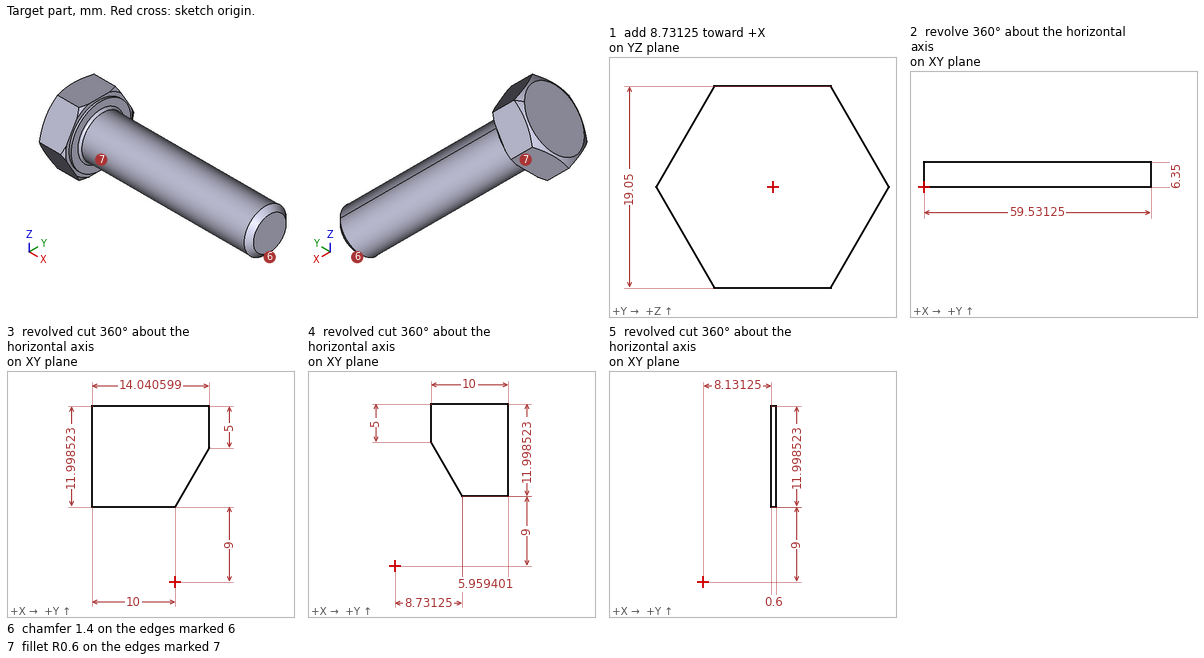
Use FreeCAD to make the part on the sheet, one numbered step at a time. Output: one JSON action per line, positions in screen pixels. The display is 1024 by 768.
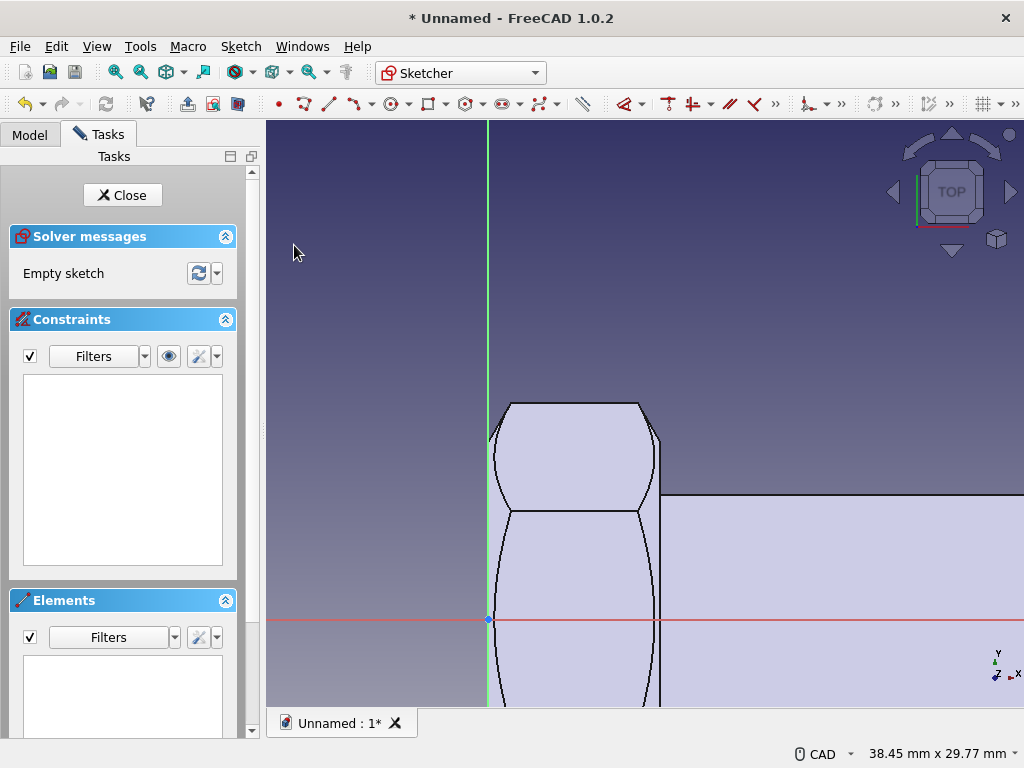
{"action": "left_click", "coordinate": [428, 104]}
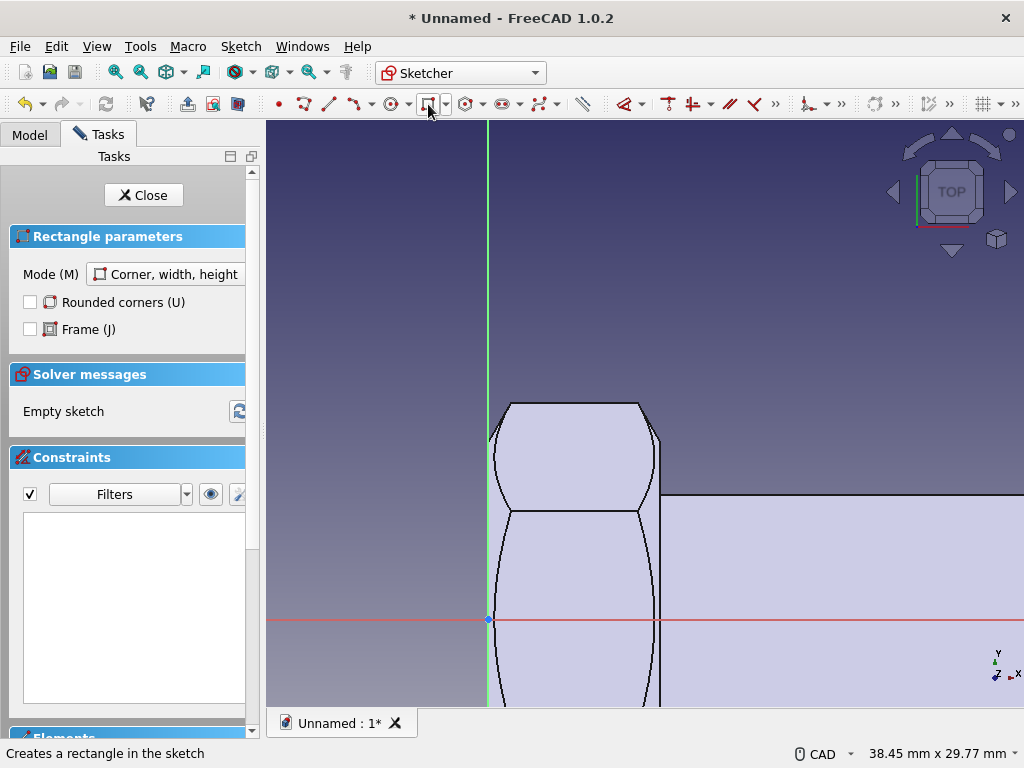
{"action": "scroll", "coordinate": [649, 206], "scroll_direction": "up", "scroll_amount": 2}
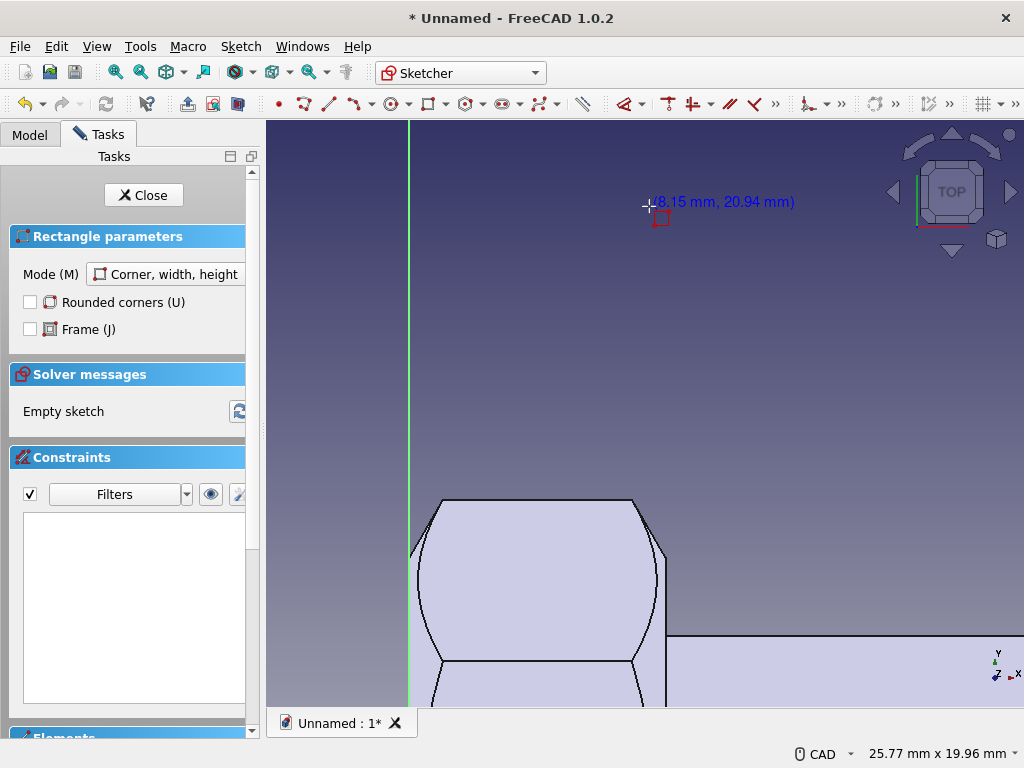
{"action": "left_click", "coordinate": [648, 206]}
{"action": "left_click", "coordinate": [666, 558]}
{"action": "key", "text": "Escape"}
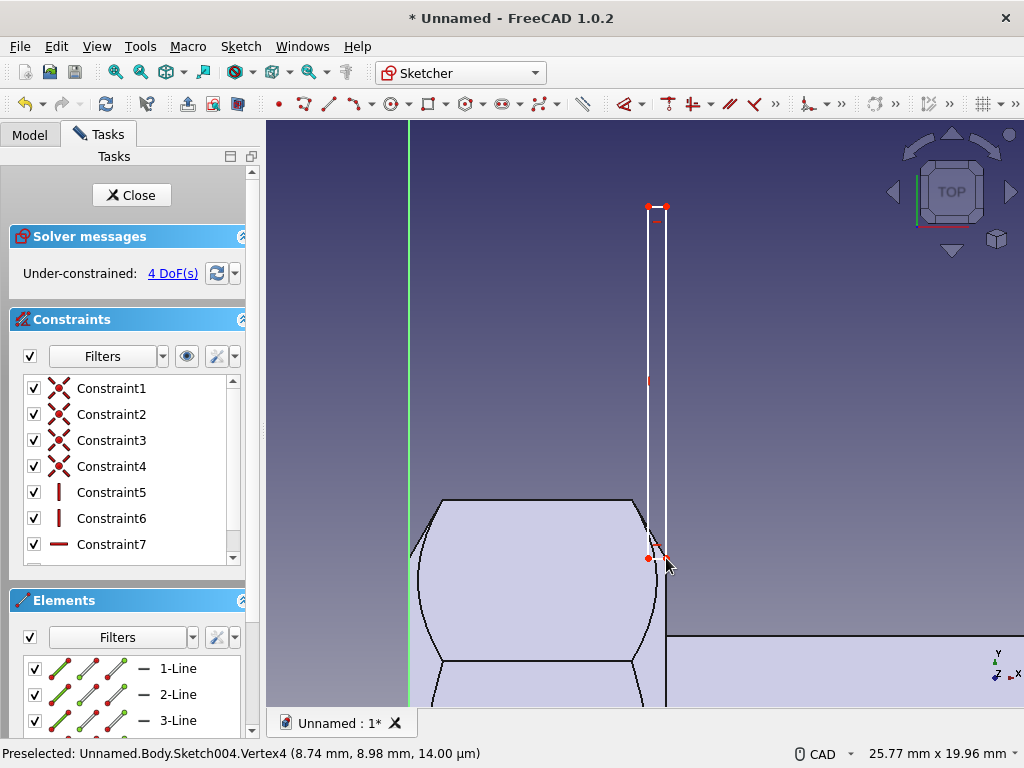
{"action": "left_click", "coordinate": [624, 104]}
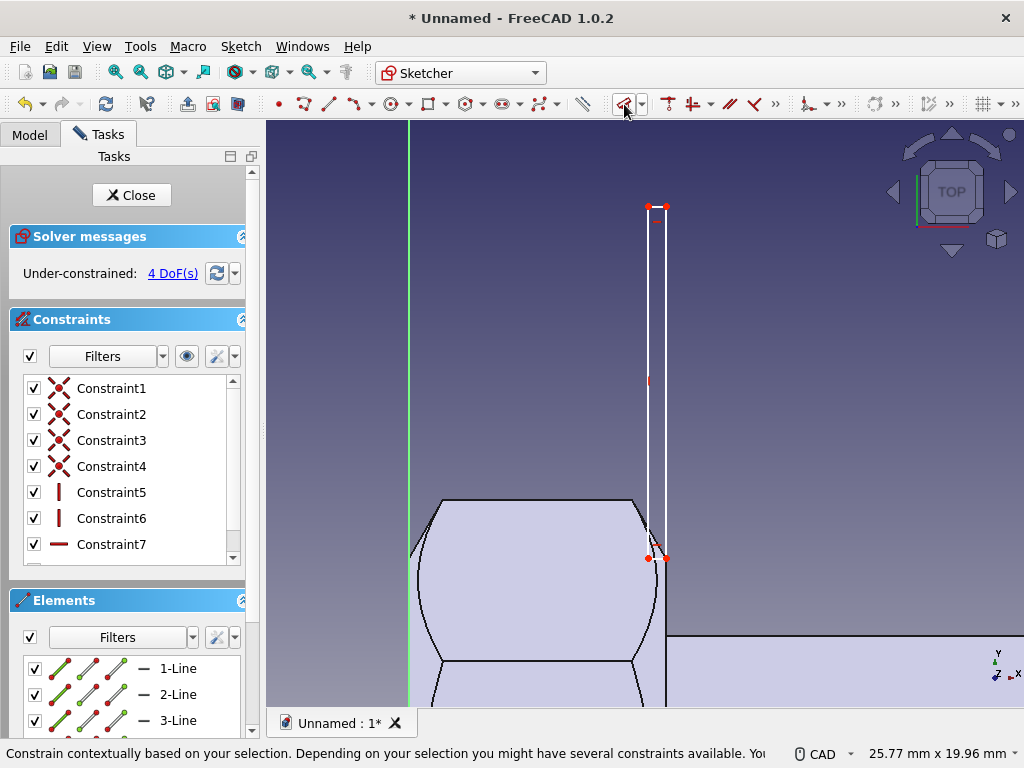
{"action": "left_click", "coordinate": [648, 559]}
{"action": "left_click", "coordinate": [375, 619]}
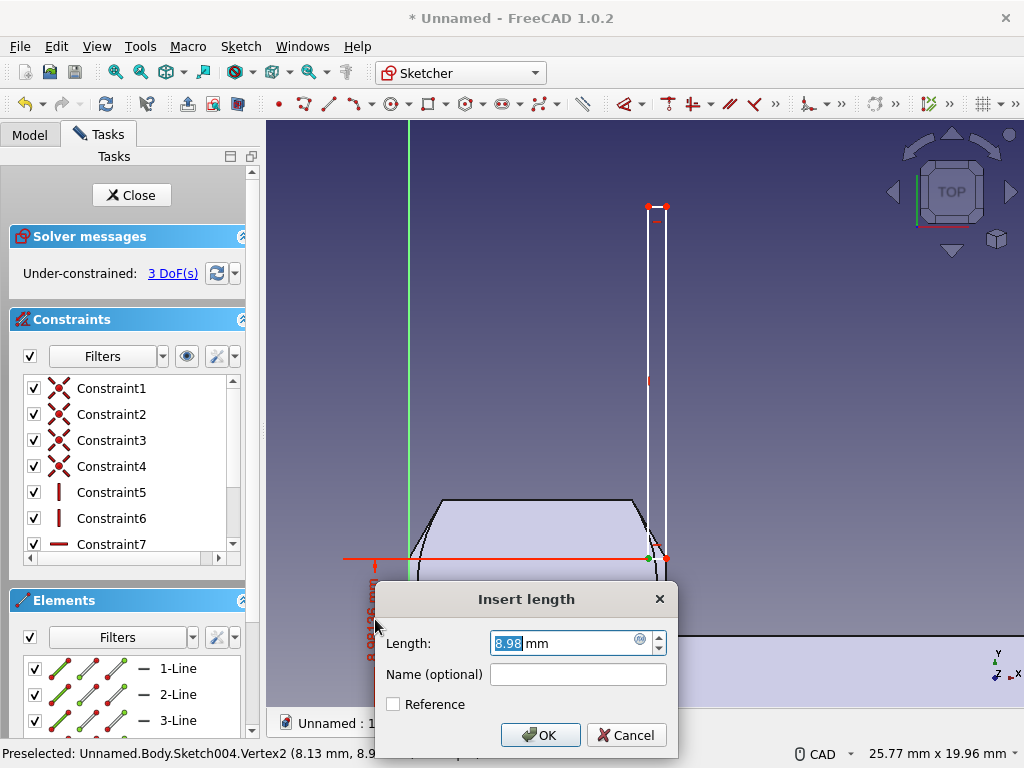
{"action": "type", "text": "9"}
{"action": "key", "text": "Return"}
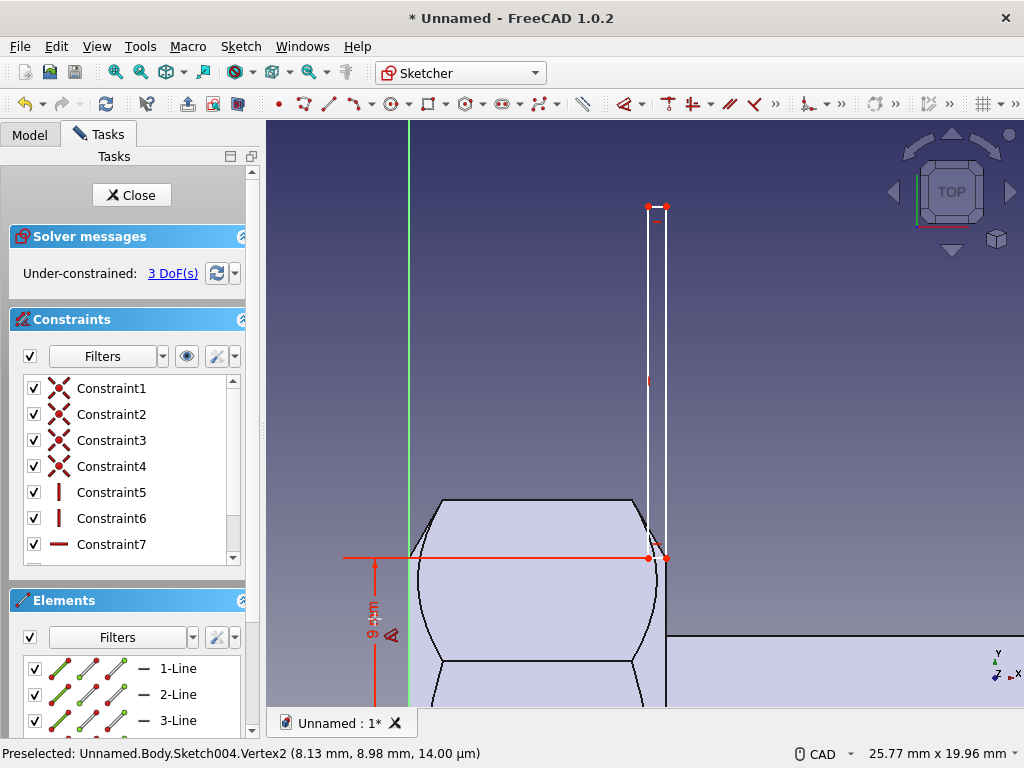
{"action": "scroll", "coordinate": [657, 558], "scroll_direction": "up", "scroll_amount": 5}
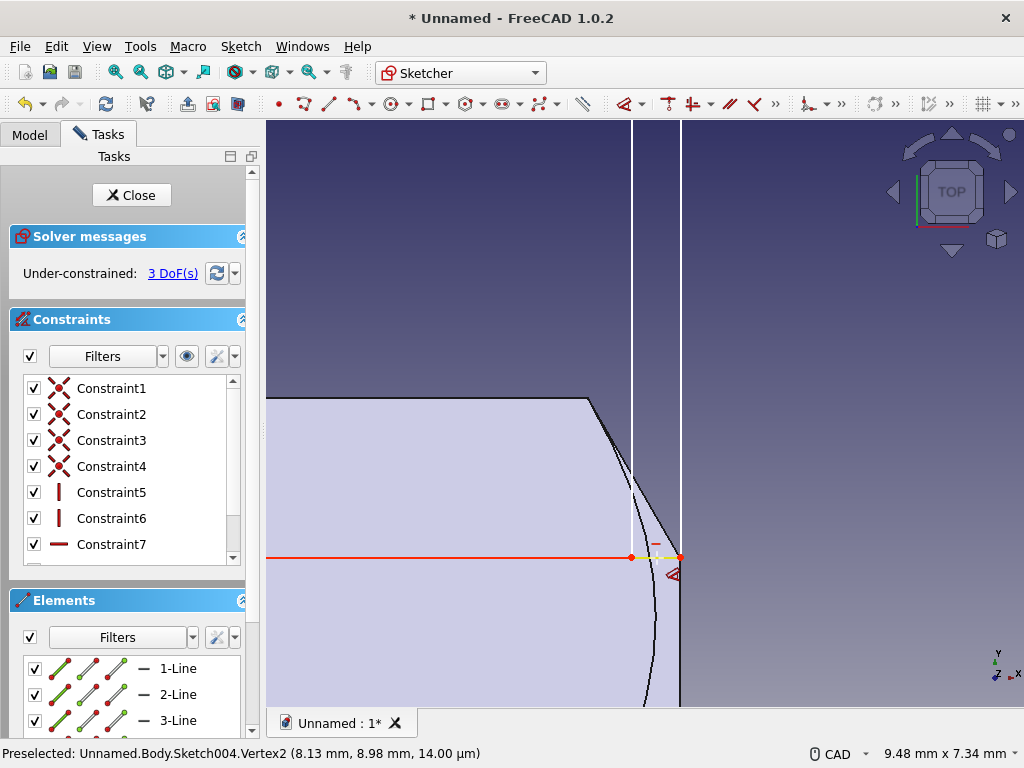
{"action": "left_click", "coordinate": [656, 558]}
{"action": "left_click", "coordinate": [656, 592]}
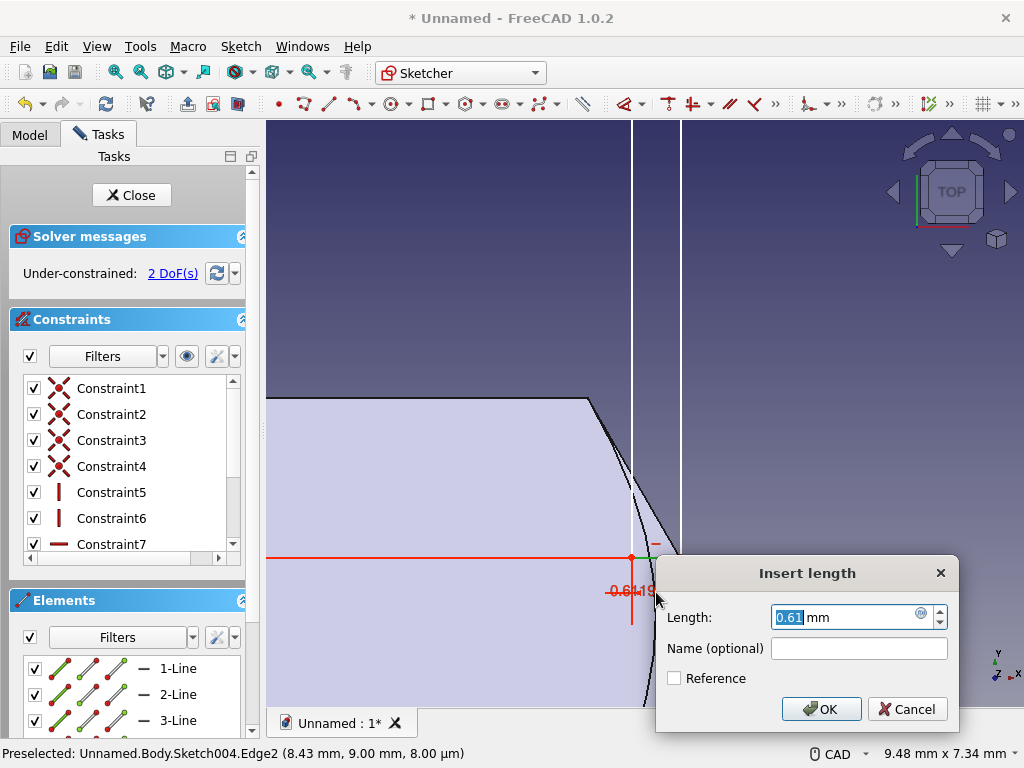
{"action": "type", "text": "0.6"}
{"action": "key", "text": "Return"}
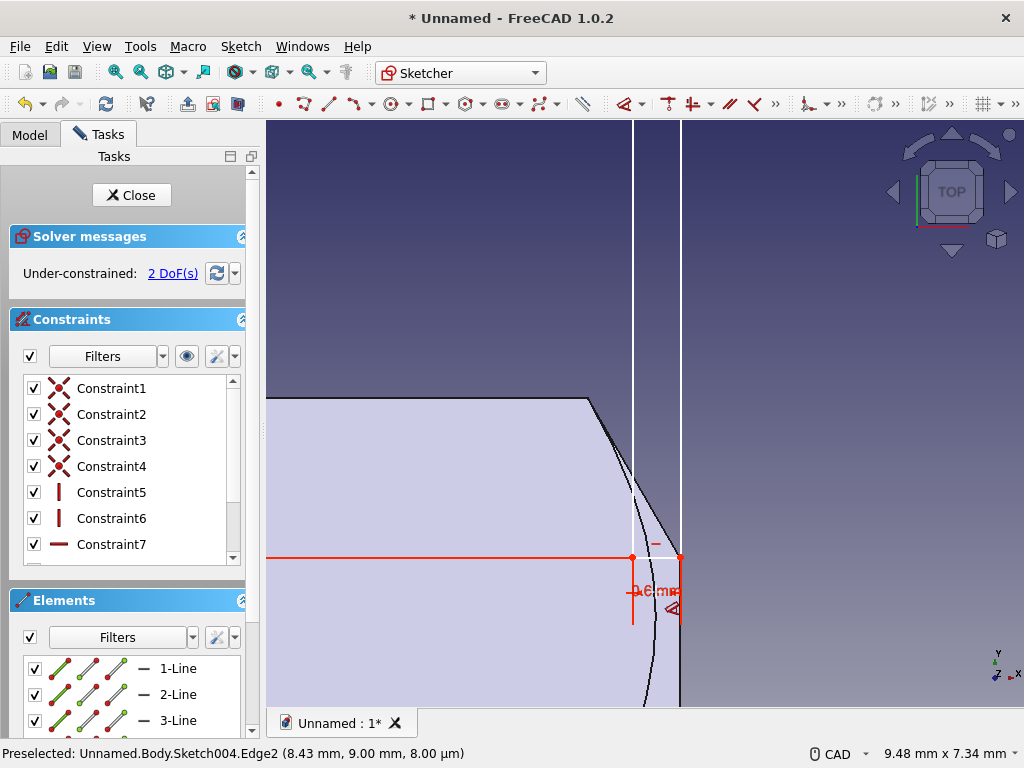
{"action": "scroll", "coordinate": [657, 405], "scroll_direction": "down", "scroll_amount": 7}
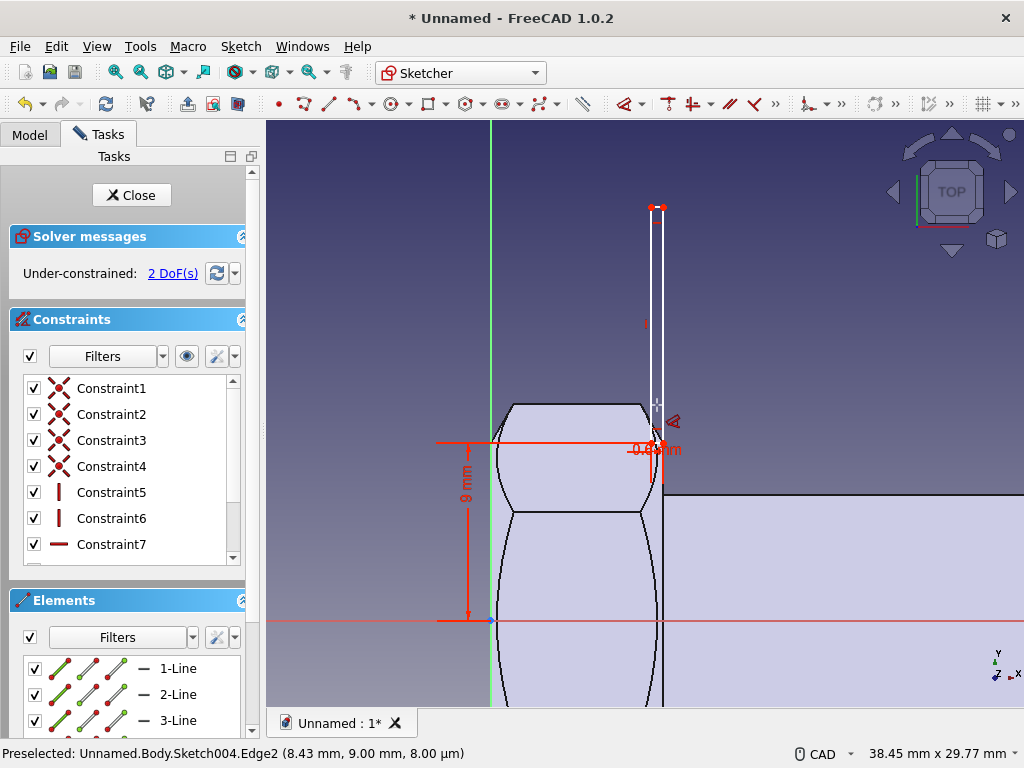
{"action": "left_click", "coordinate": [651, 207]}
{"action": "left_click", "coordinate": [571, 655]}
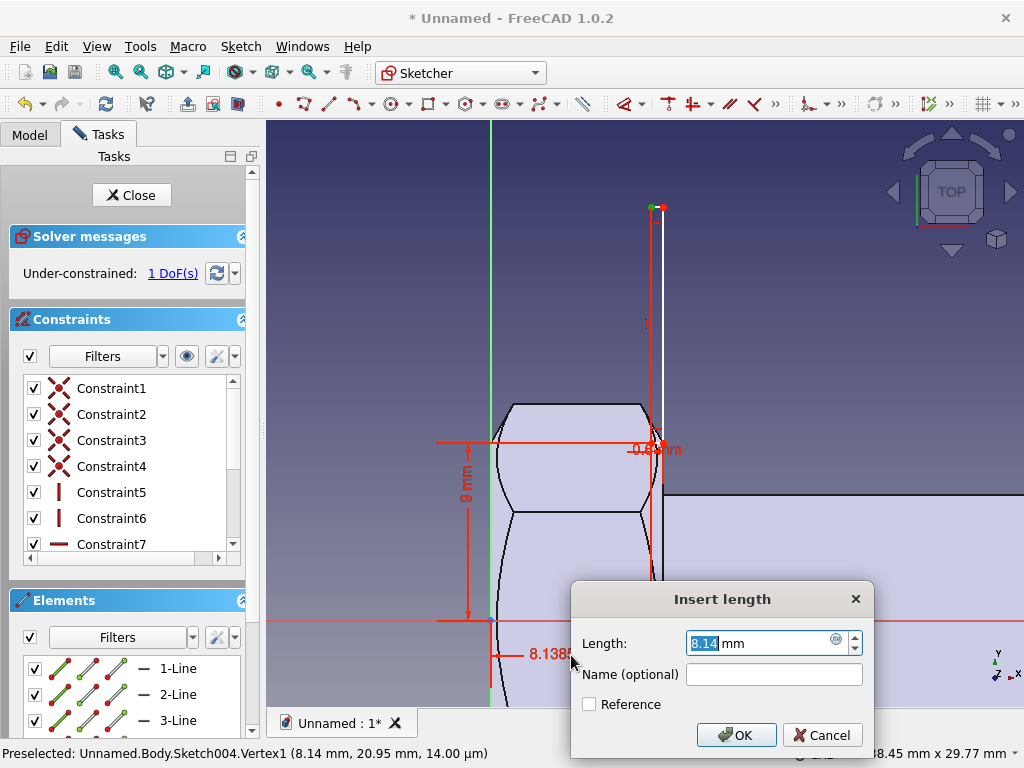
{"action": "type", "text": "8.13125"}
{"action": "key", "text": "Return"}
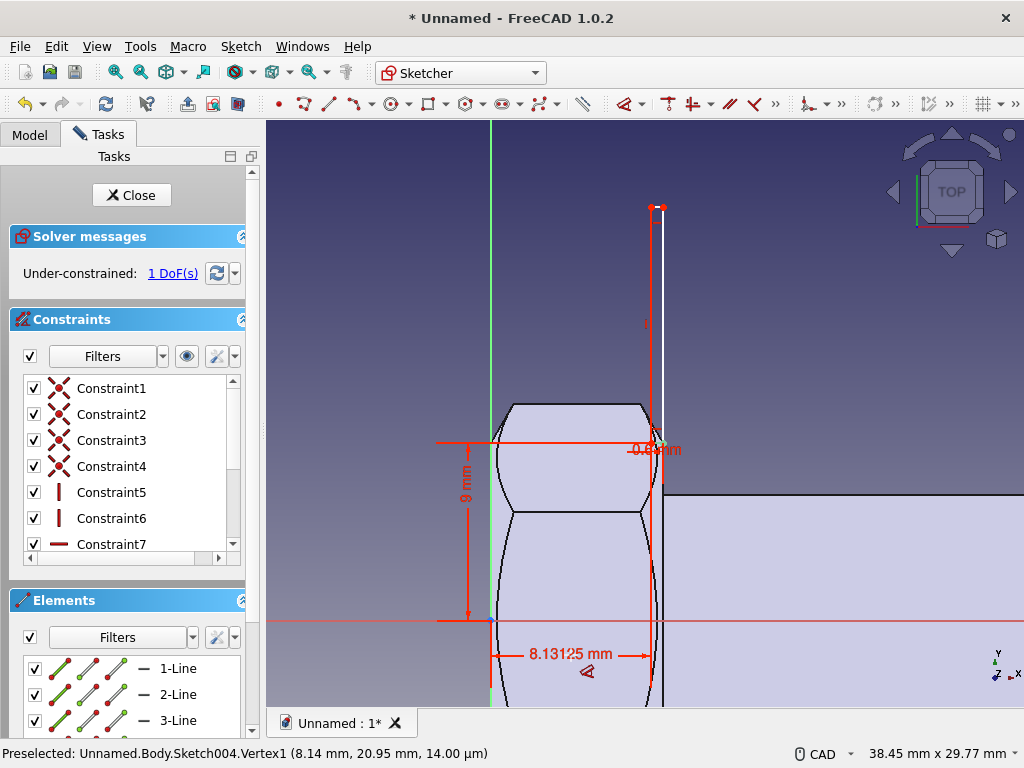
{"action": "left_click", "coordinate": [651, 278]}
{"action": "left_click", "coordinate": [685, 325]}